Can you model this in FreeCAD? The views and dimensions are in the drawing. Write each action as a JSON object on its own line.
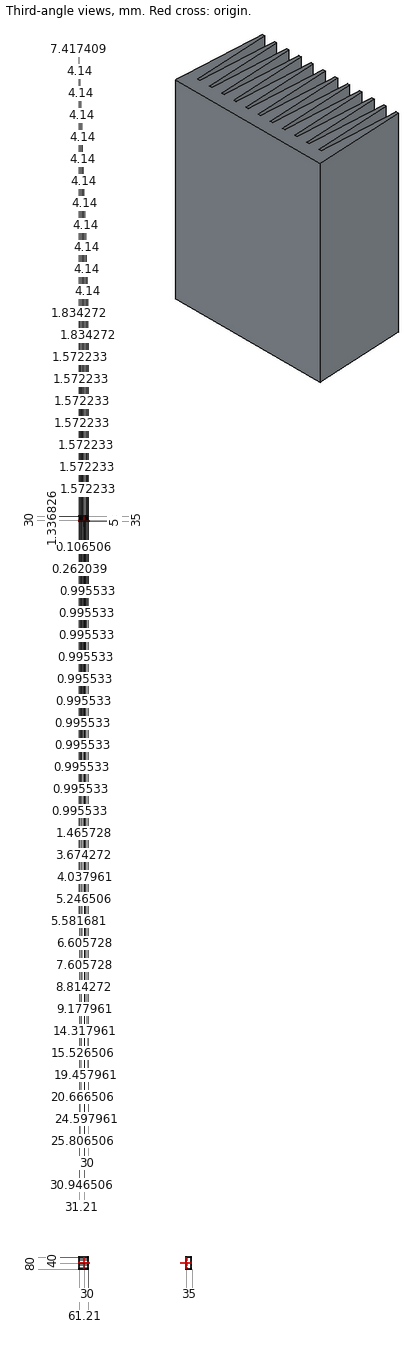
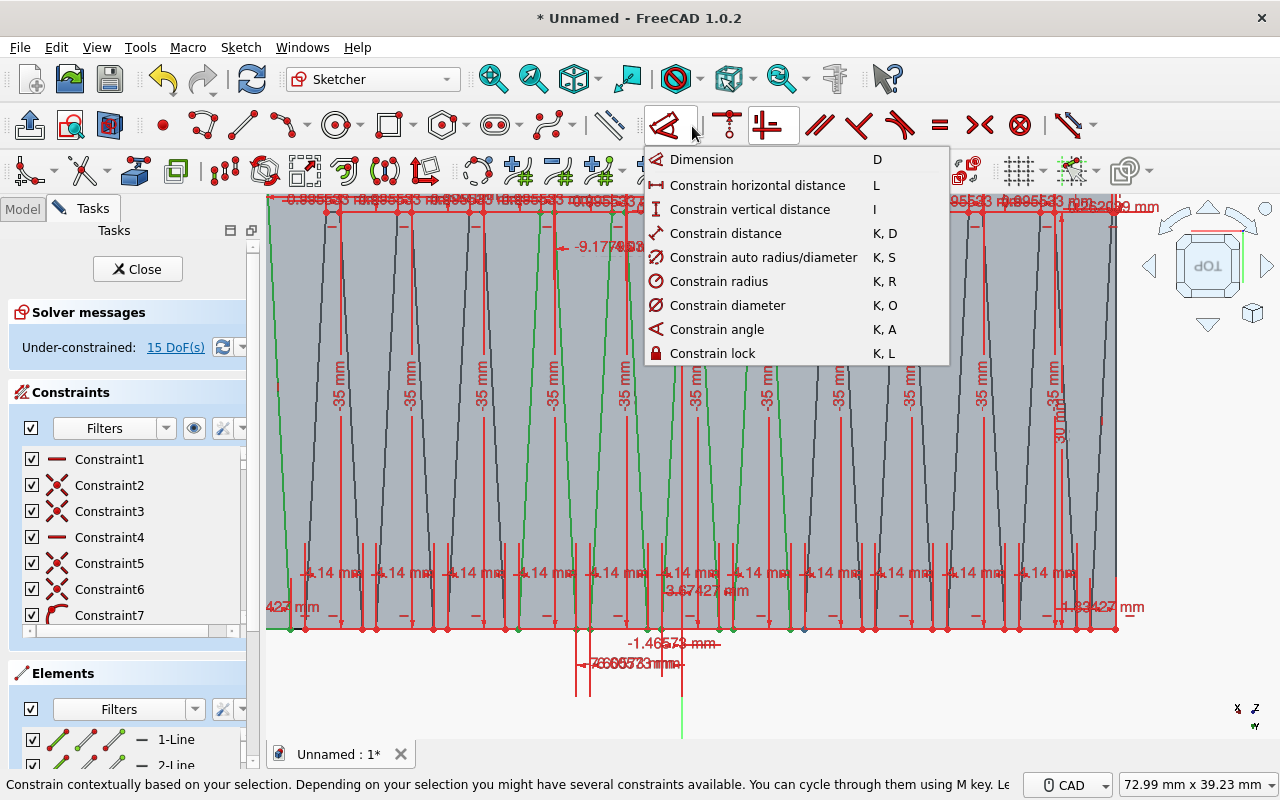
{"action": "left_click", "coordinate": [797, 185]}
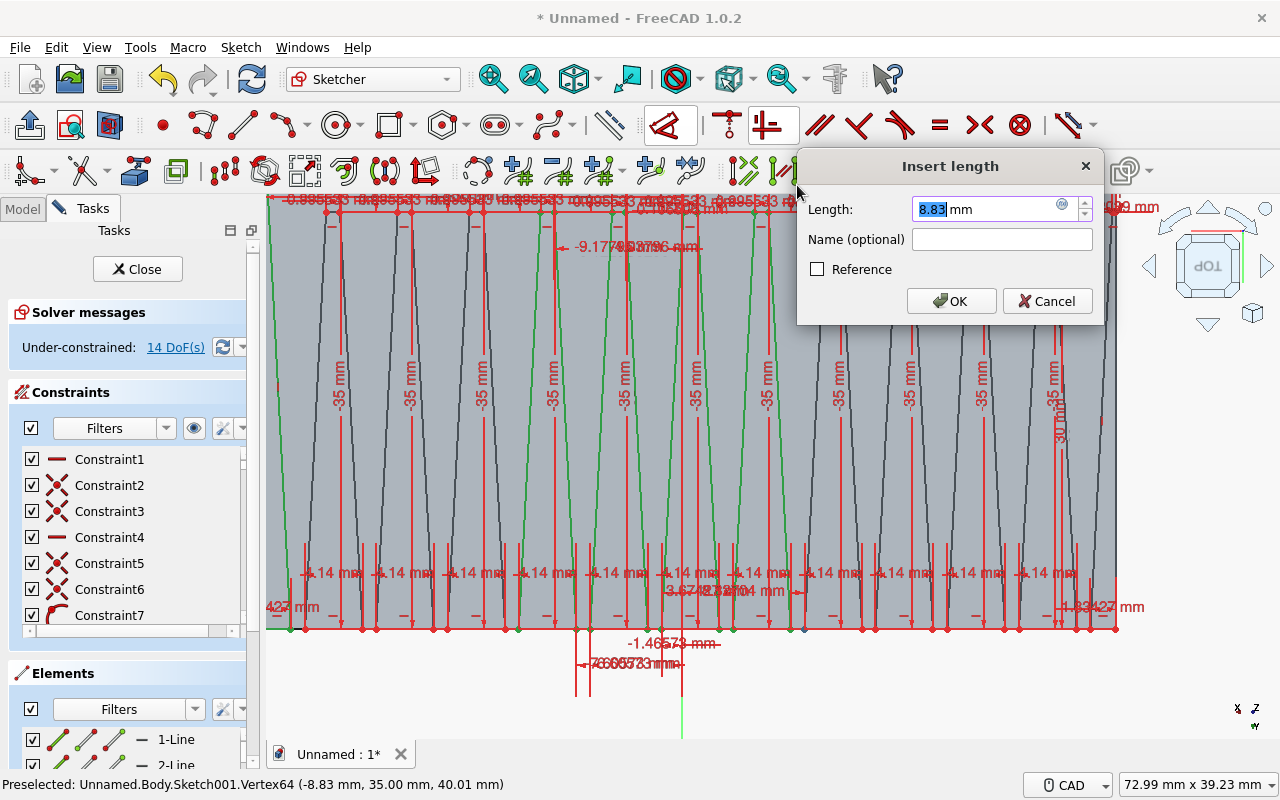
{"action": "type", "text": "8.814272"}
{"action": "key", "text": "Return"}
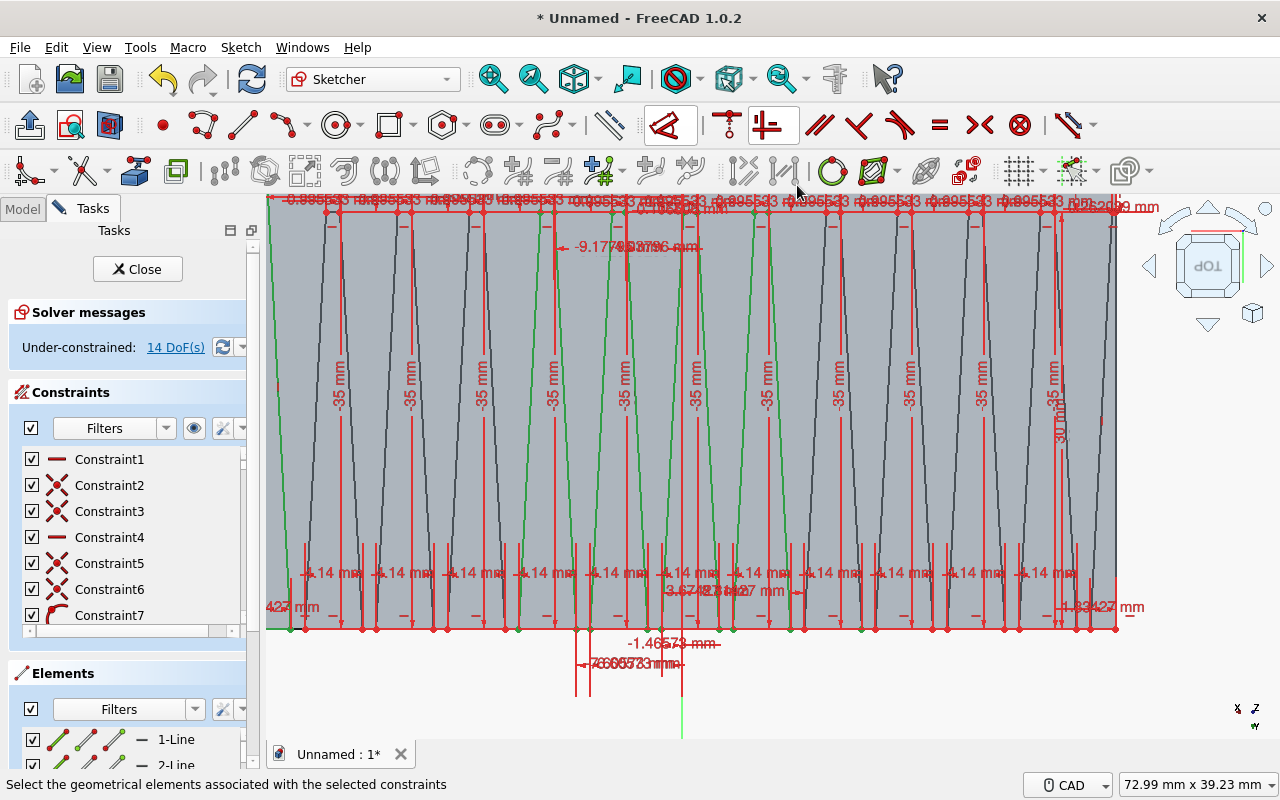
{"action": "scroll", "coordinate": [320, 337], "scroll_direction": "up", "scroll_amount": 3}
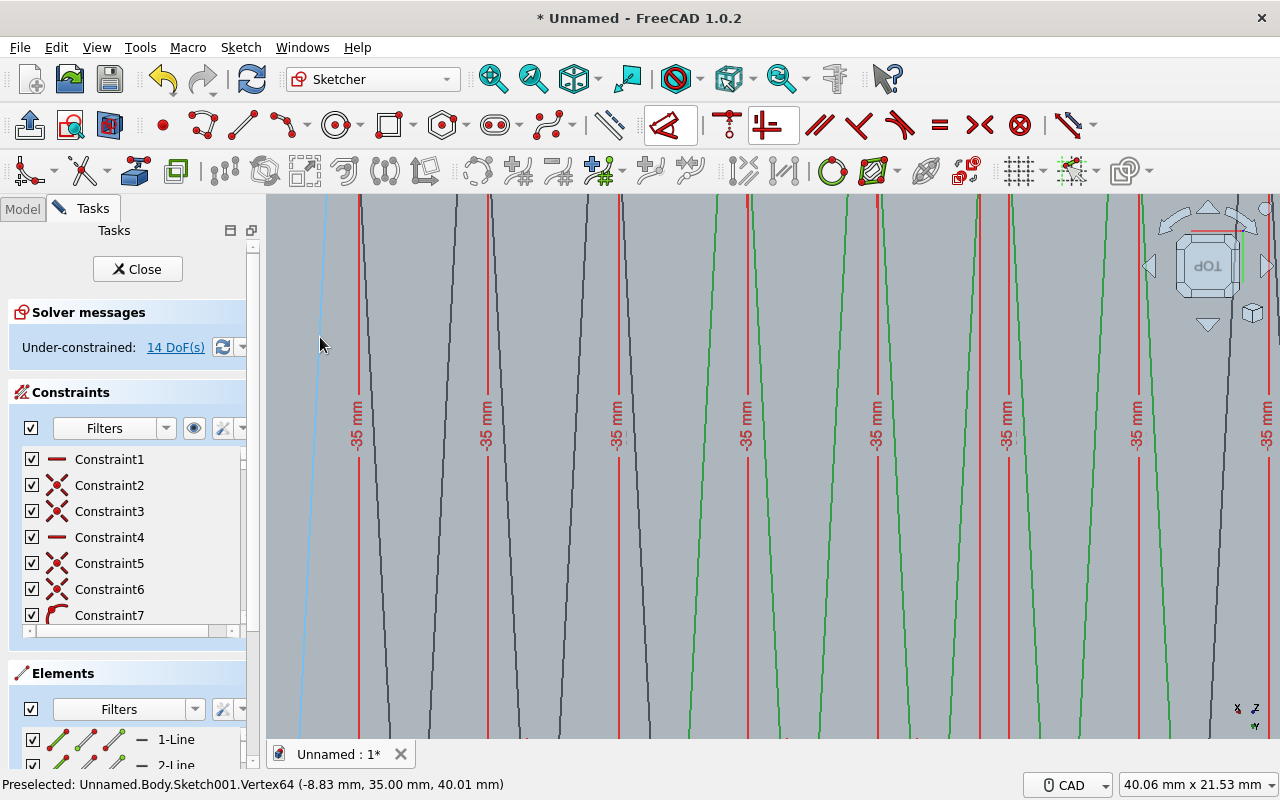
{"action": "left_click", "coordinate": [320, 338]}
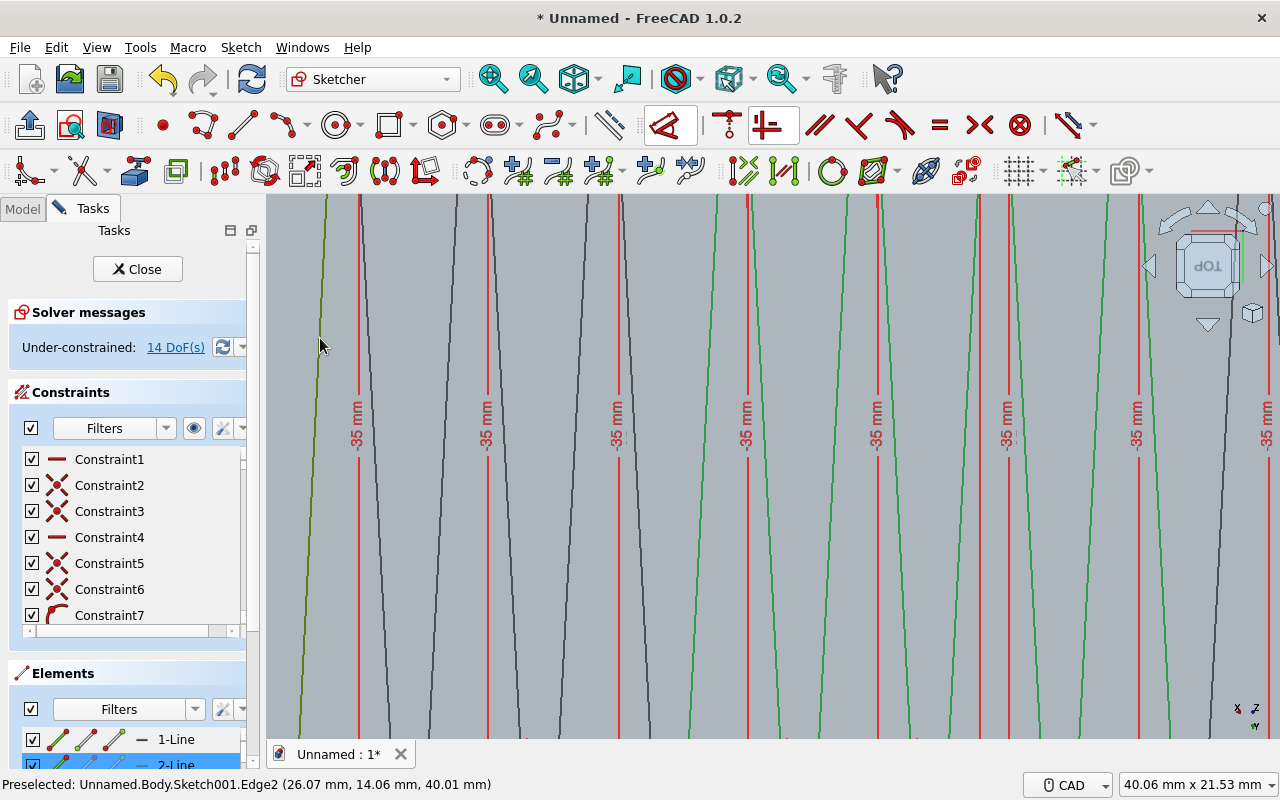
{"action": "left_click", "coordinate": [692, 126]}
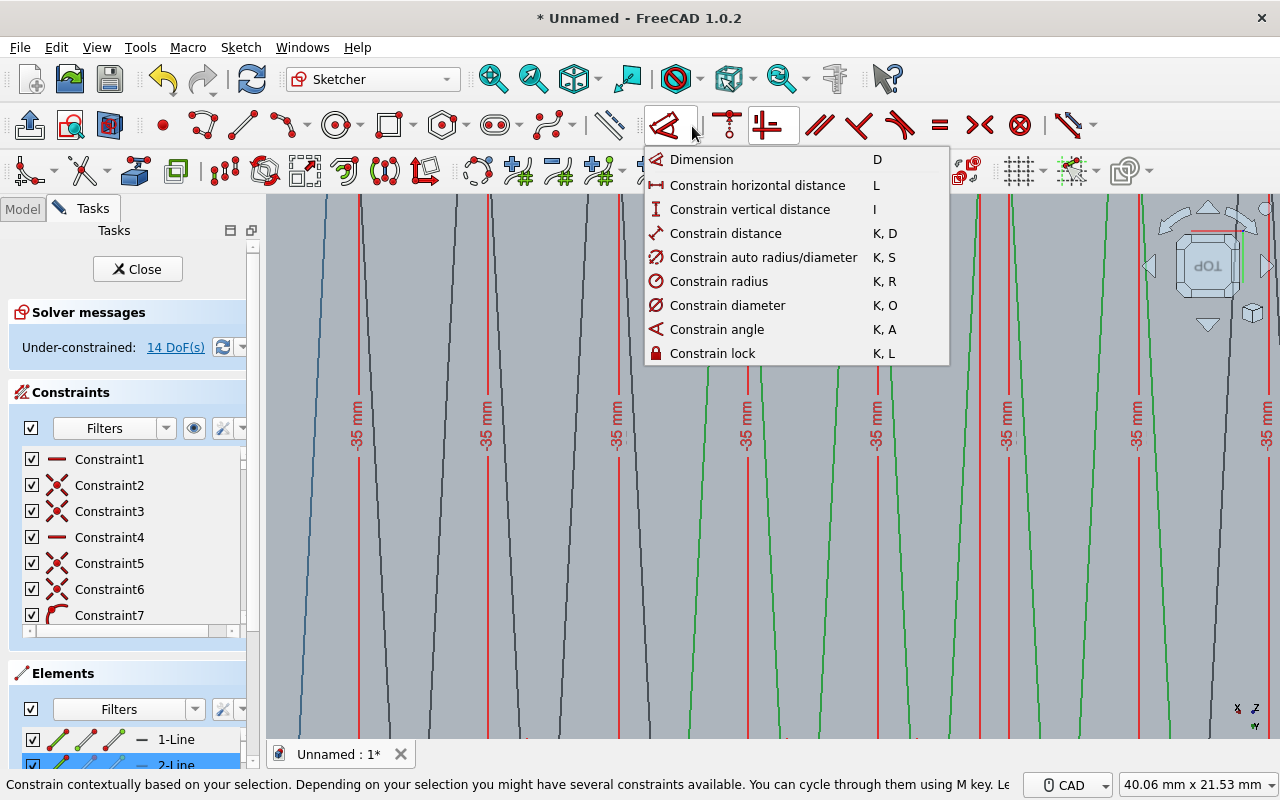
{"action": "left_click", "coordinate": [797, 185]}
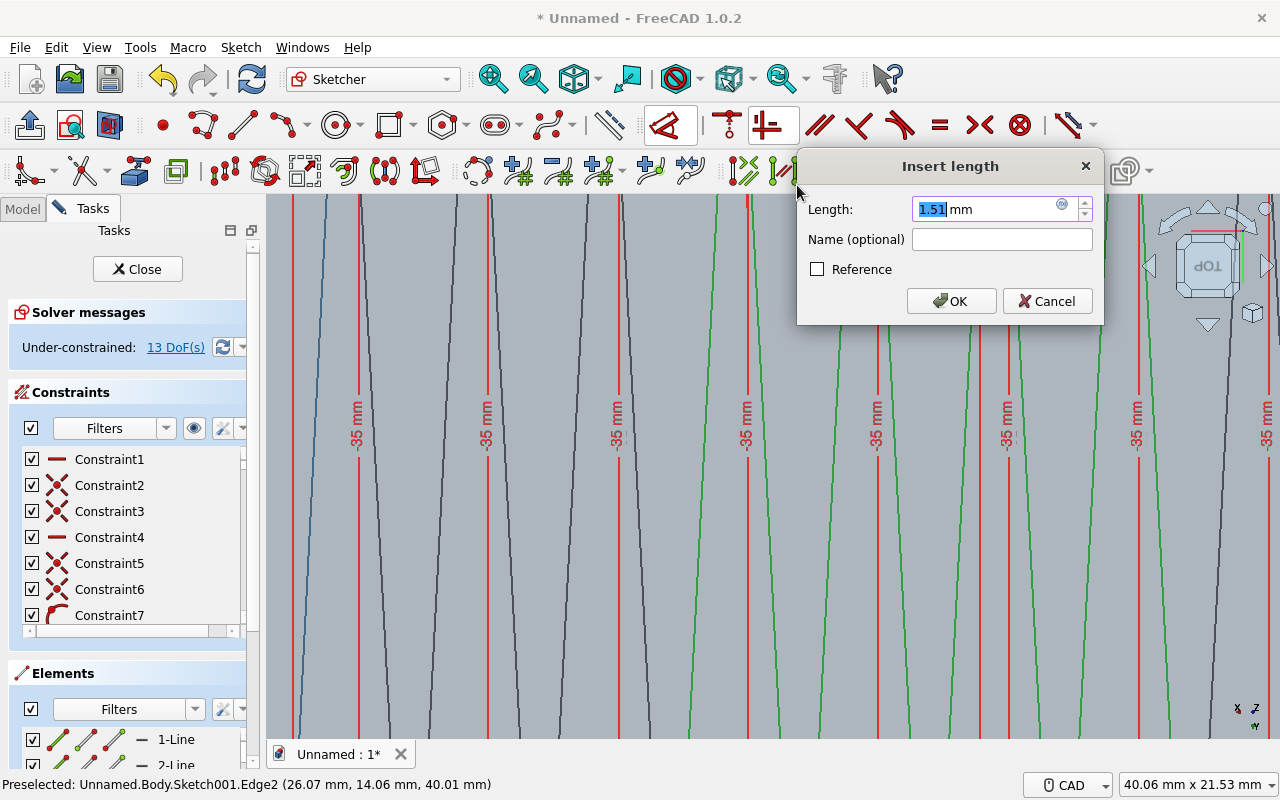
{"action": "type", "text": "1.572233"}
{"action": "key", "text": "Return"}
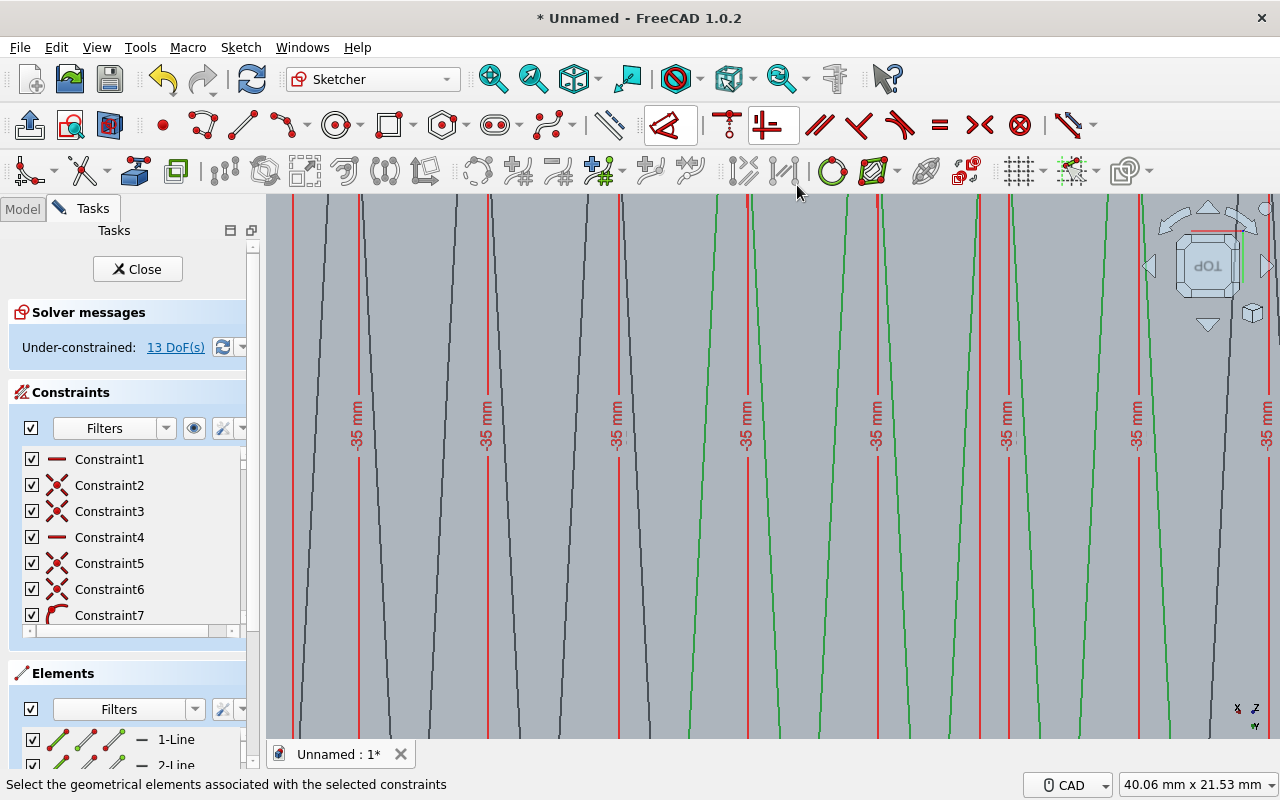
{"action": "left_click", "coordinate": [450, 338]}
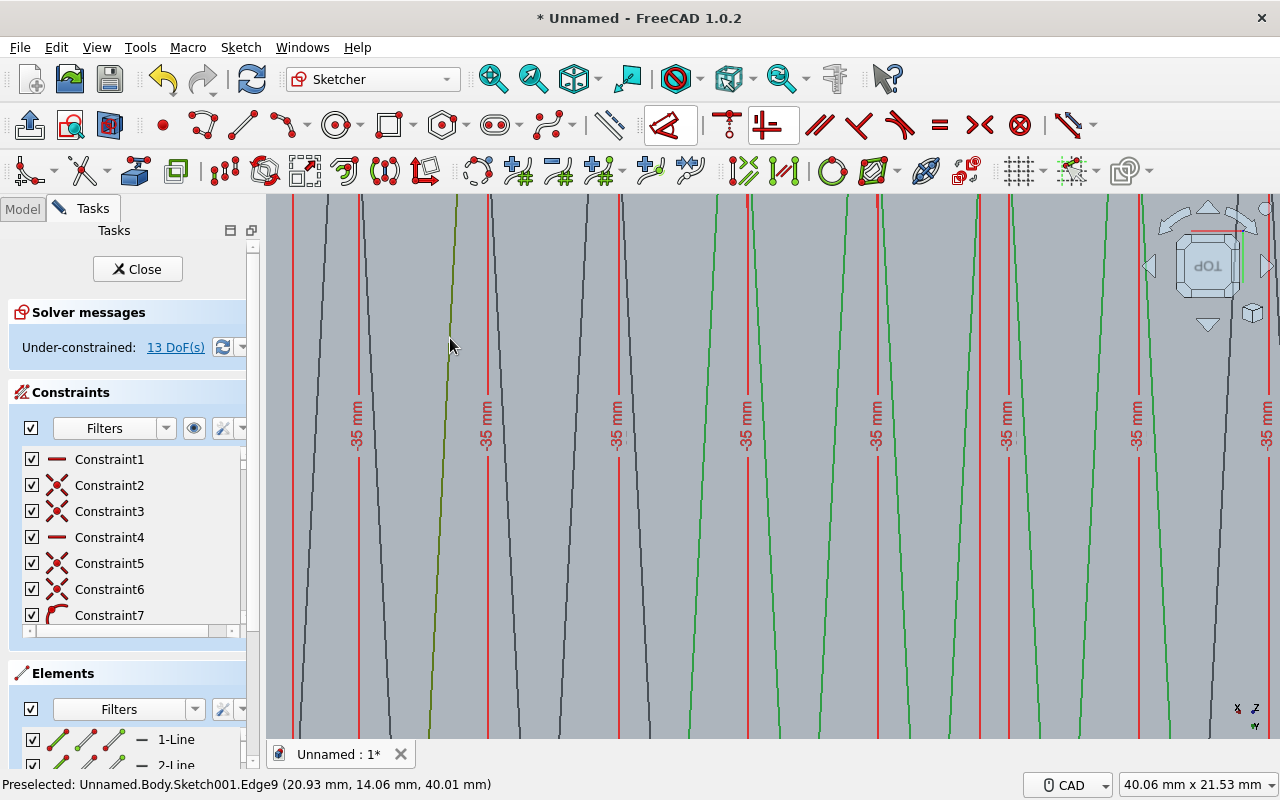
{"action": "key", "text": "l"}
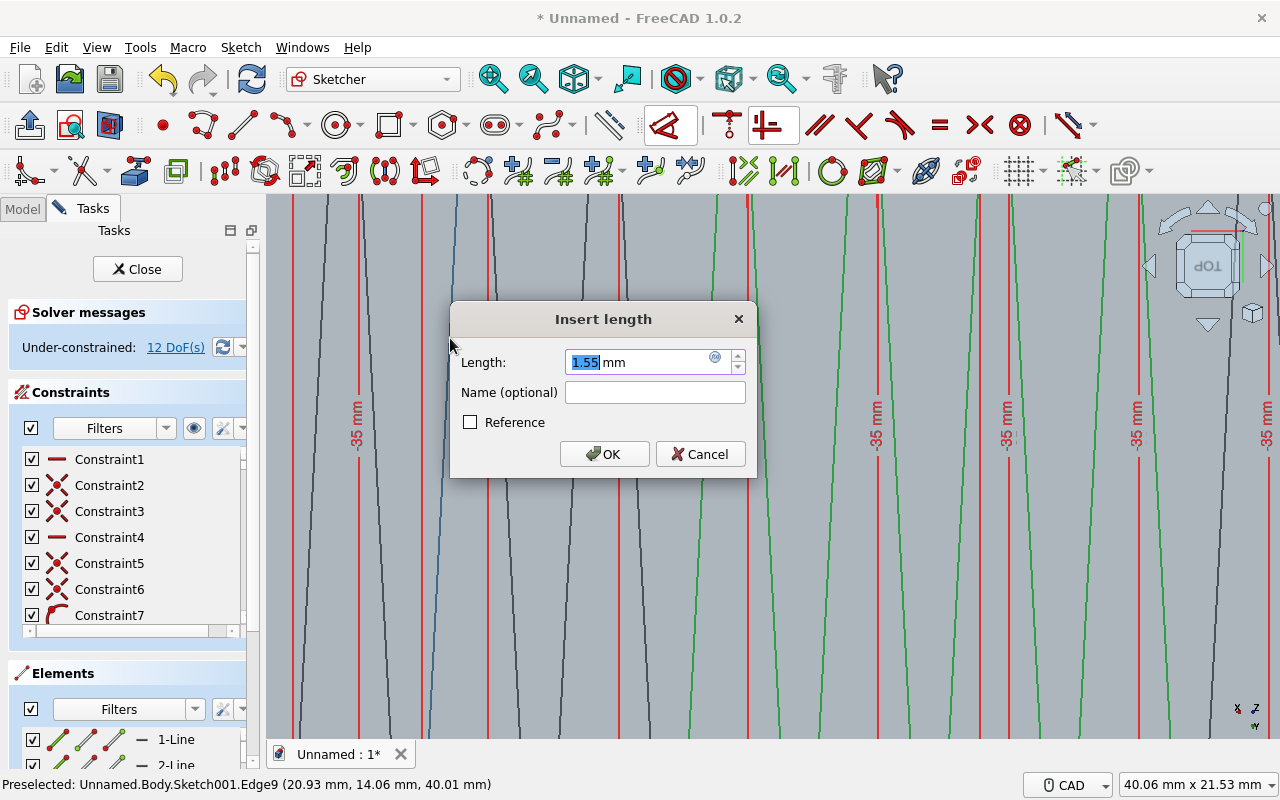
{"action": "type", "text": "1.572233"}
{"action": "key", "text": "Return"}